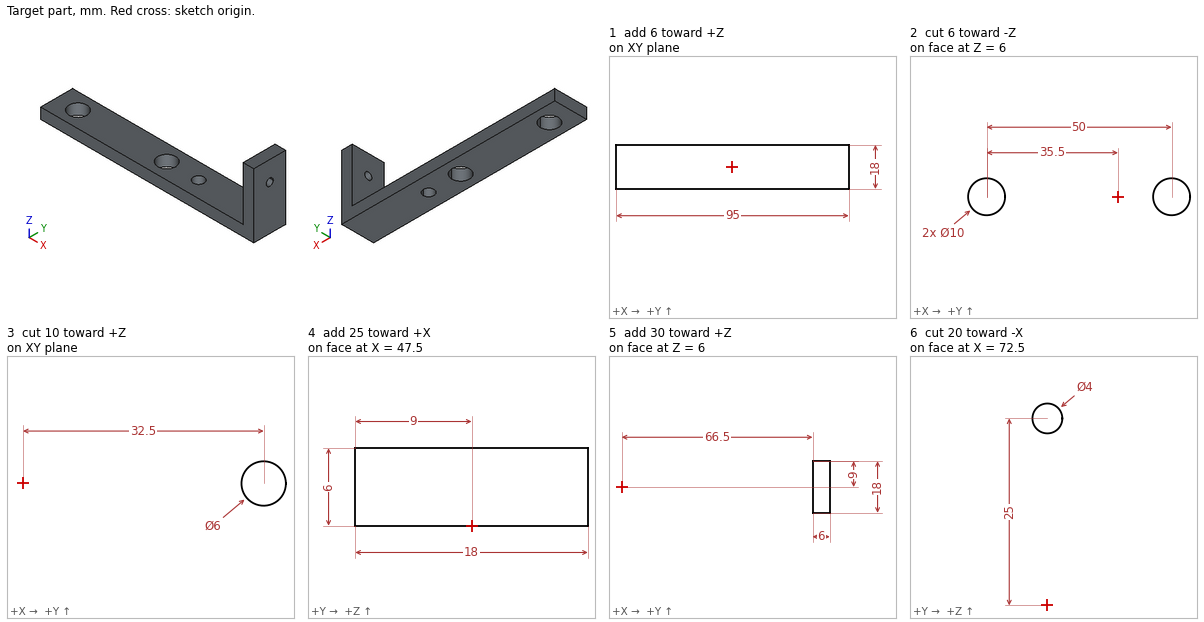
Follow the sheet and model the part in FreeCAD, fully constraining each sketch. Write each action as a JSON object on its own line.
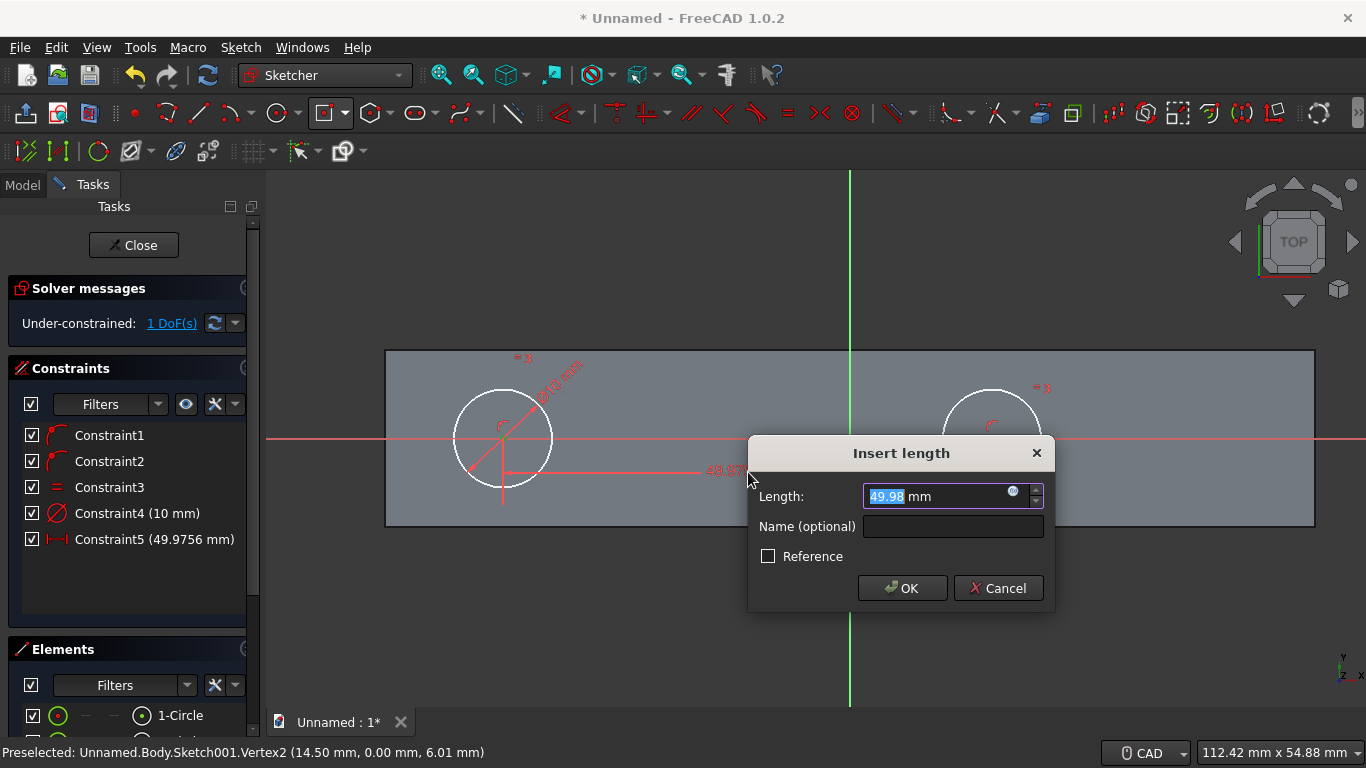
{"action": "type", "text": "50"}
{"action": "key", "text": "Return"}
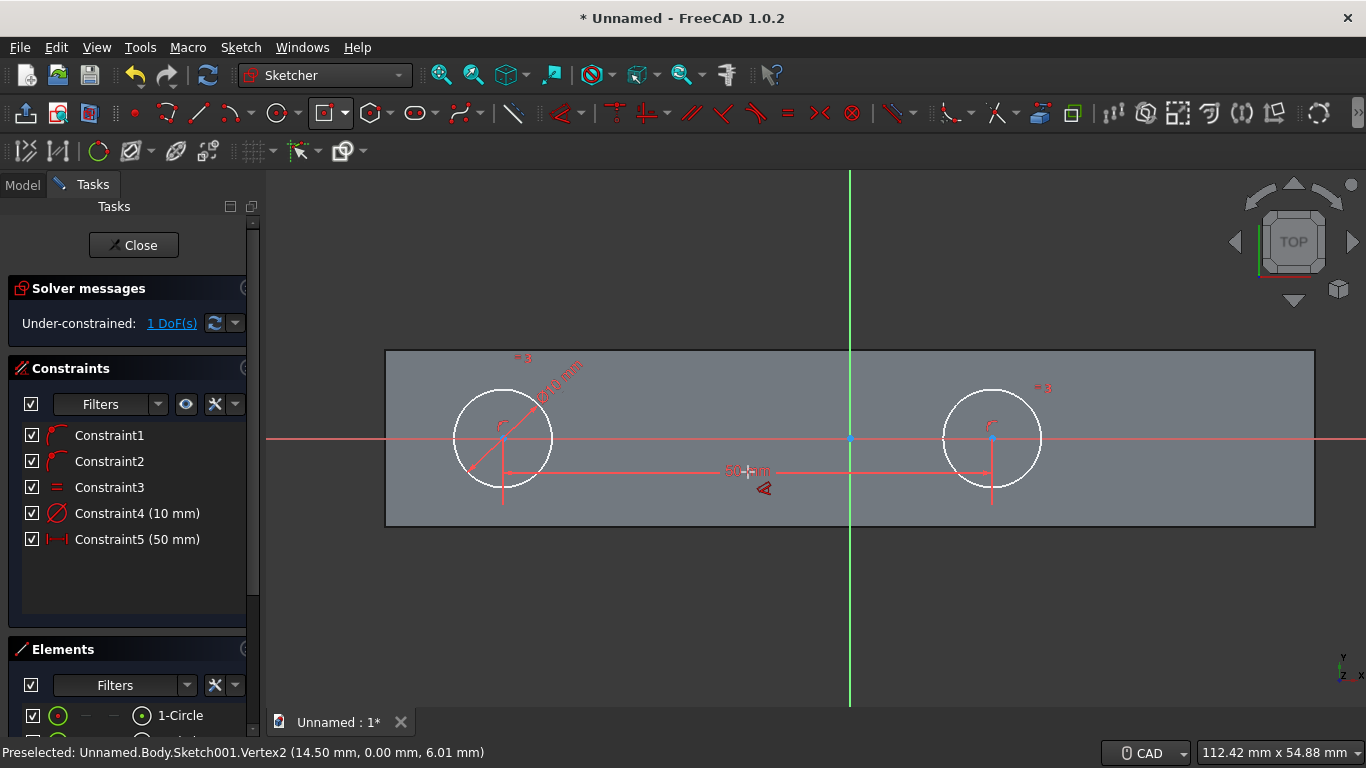
{"action": "left_click", "coordinate": [503, 438]}
{"action": "left_click", "coordinate": [677, 472]}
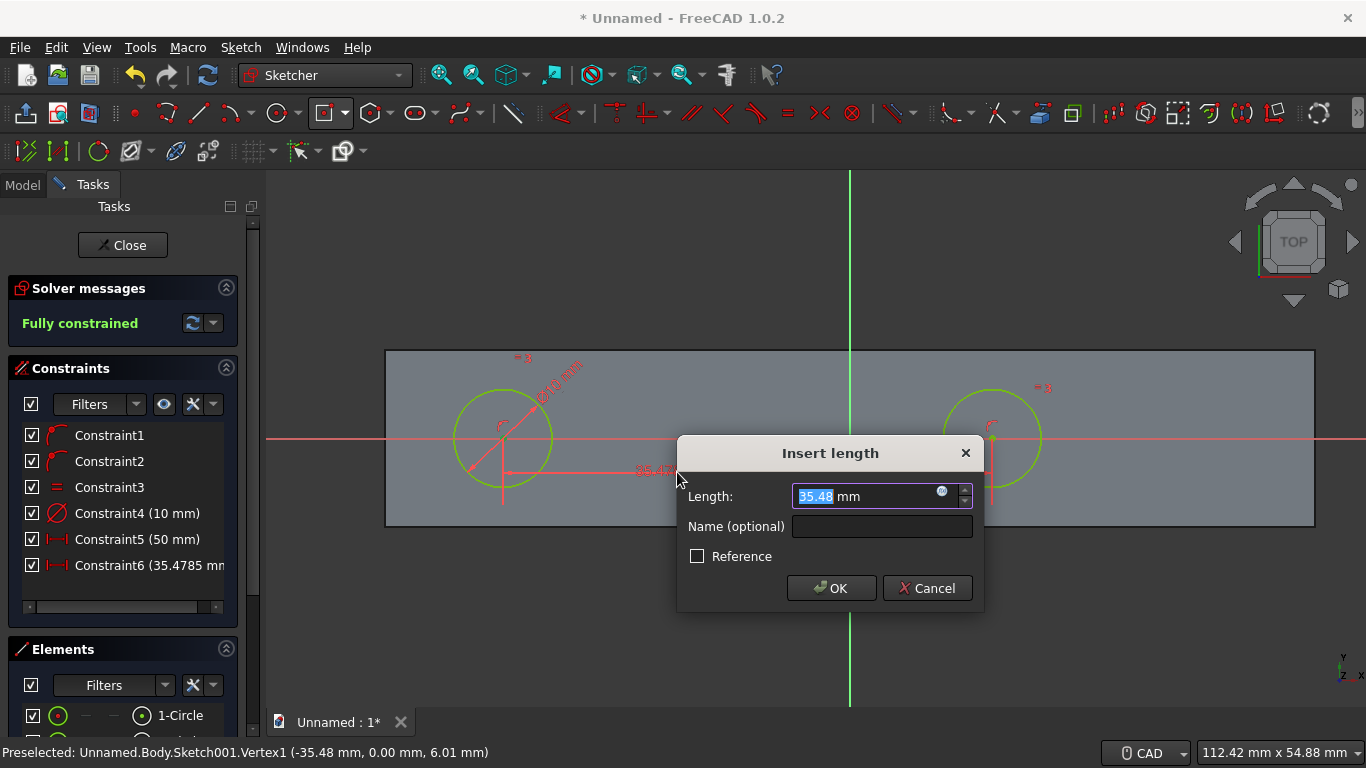
{"action": "type", "text": "35.5"}
{"action": "key", "text": "Return"}
{"action": "key", "text": "Escape"}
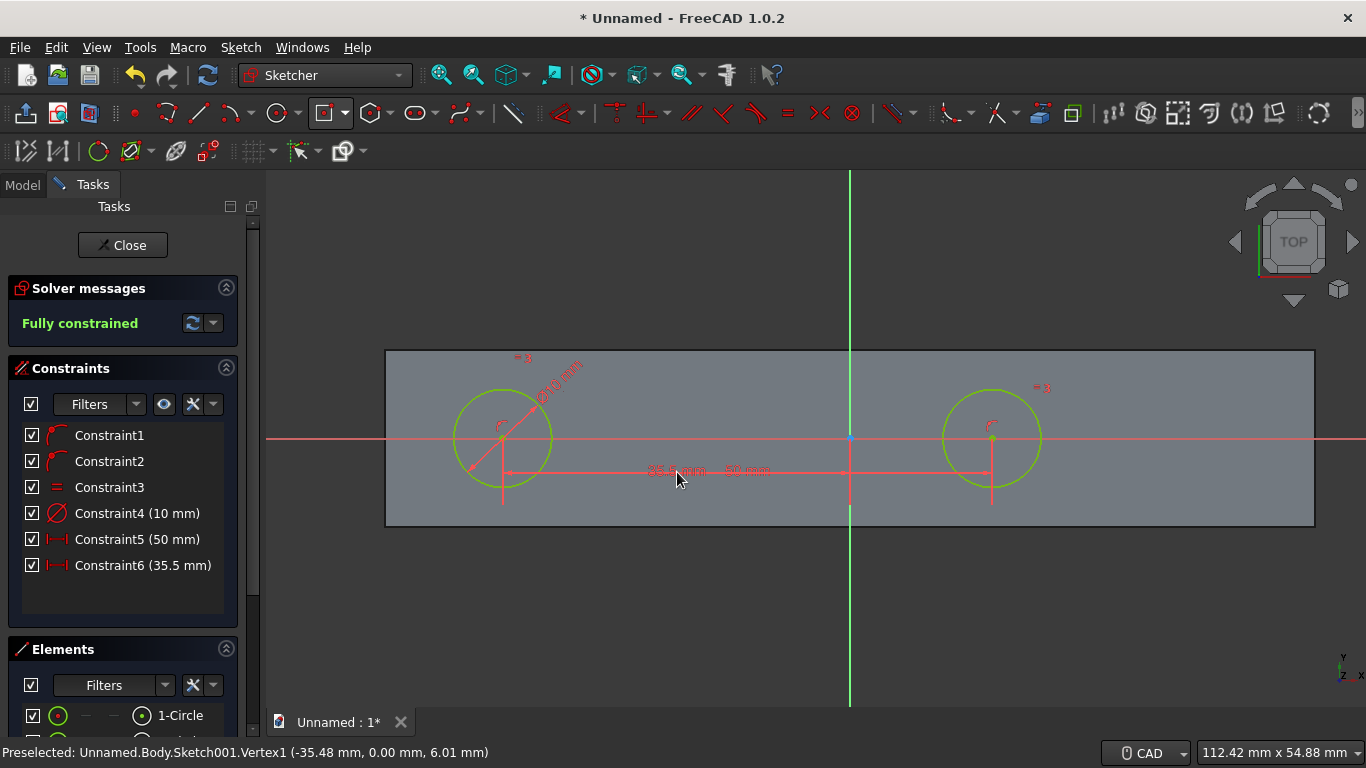
{"action": "left_click", "coordinate": [123, 245]}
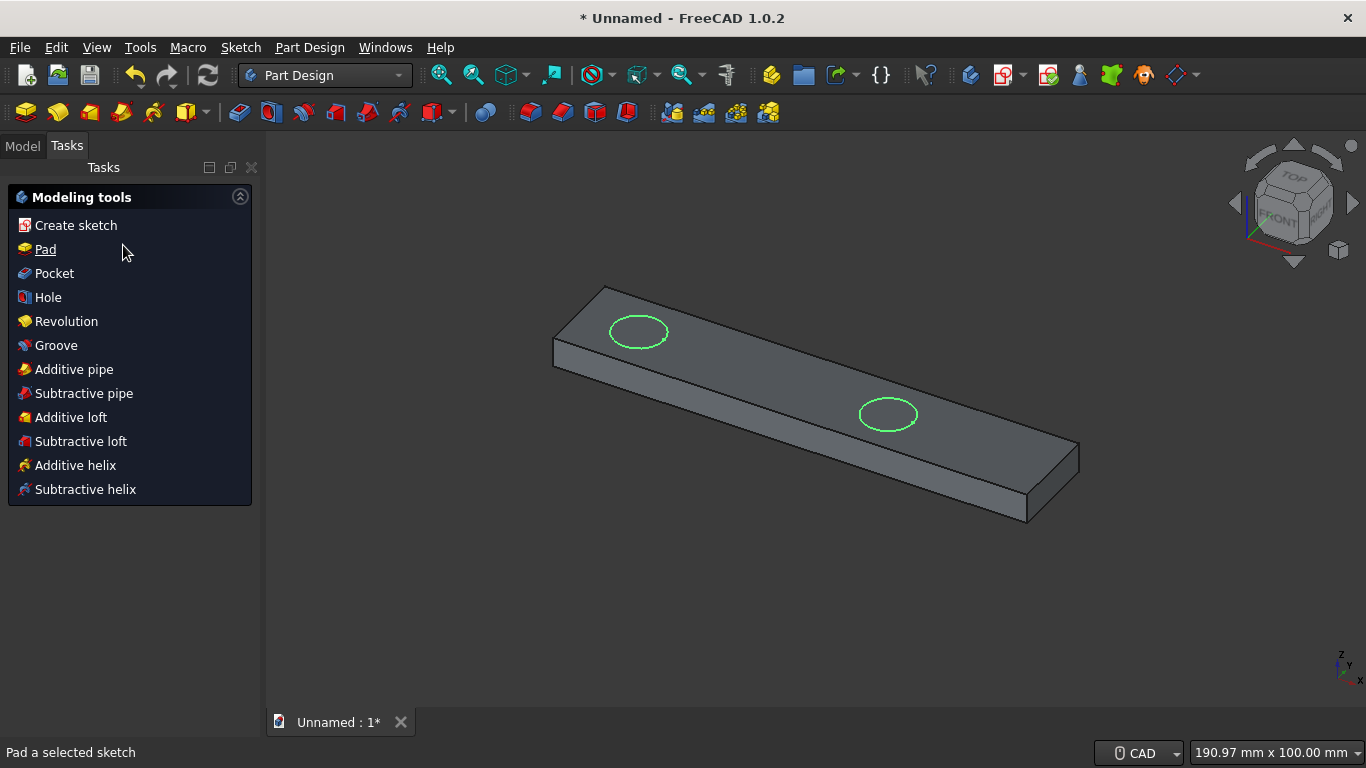
{"action": "left_click", "coordinate": [240, 112]}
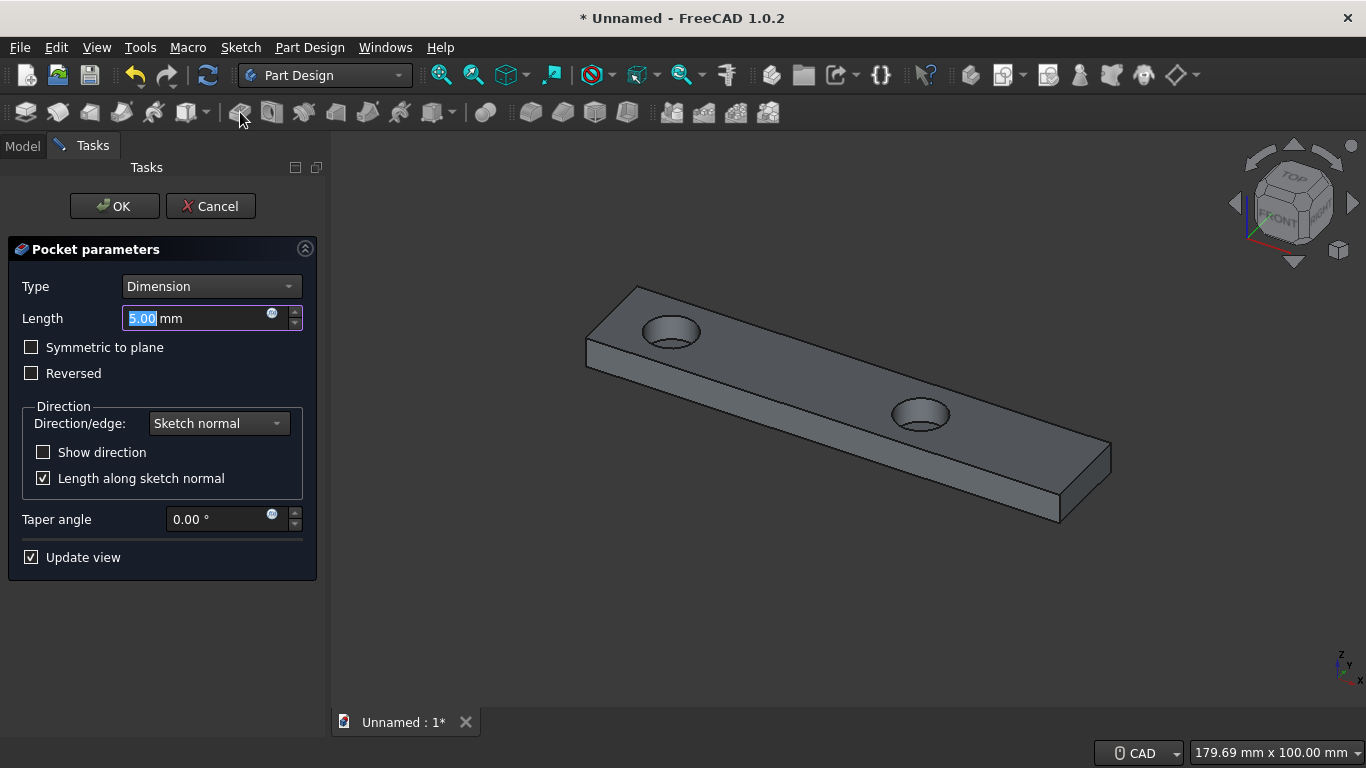
{"action": "type", "text": "6"}
{"action": "key", "text": "Tab"}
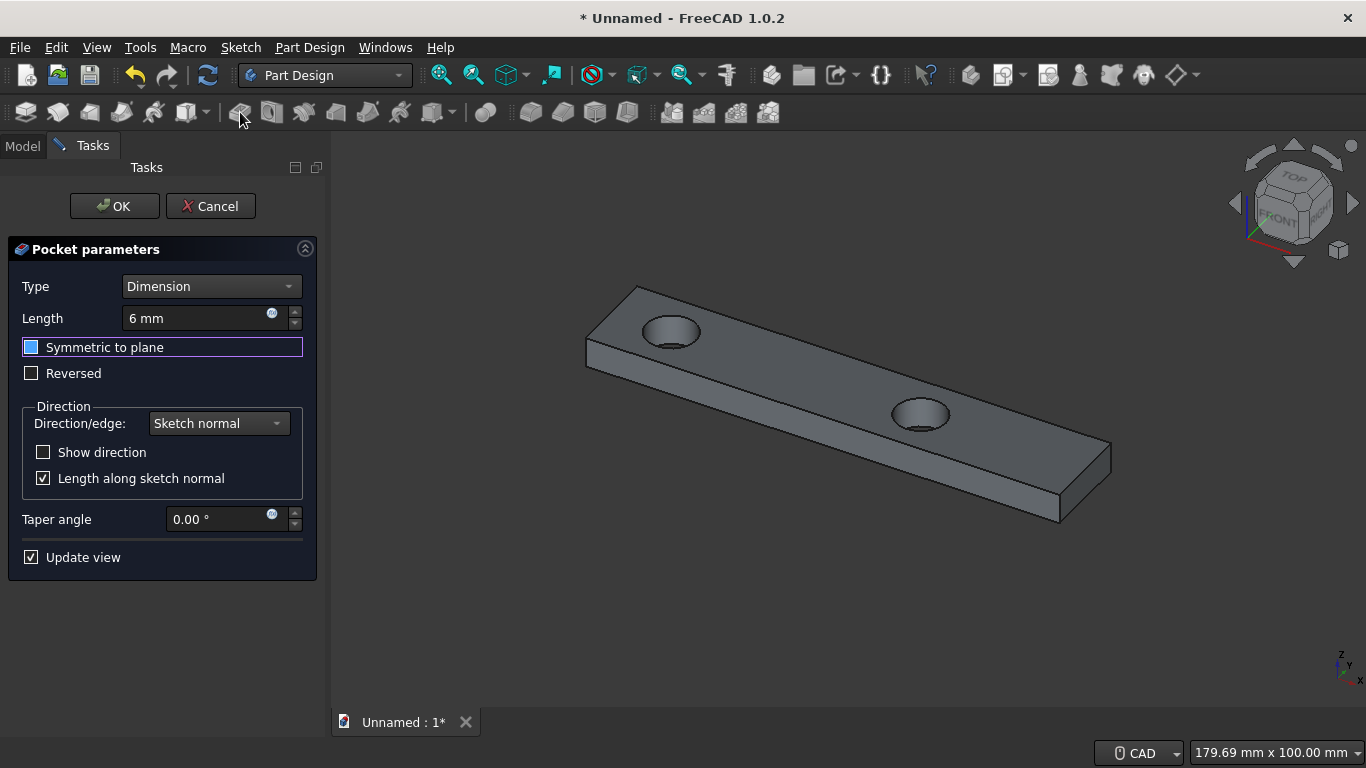
{"action": "left_click", "coordinate": [115, 206]}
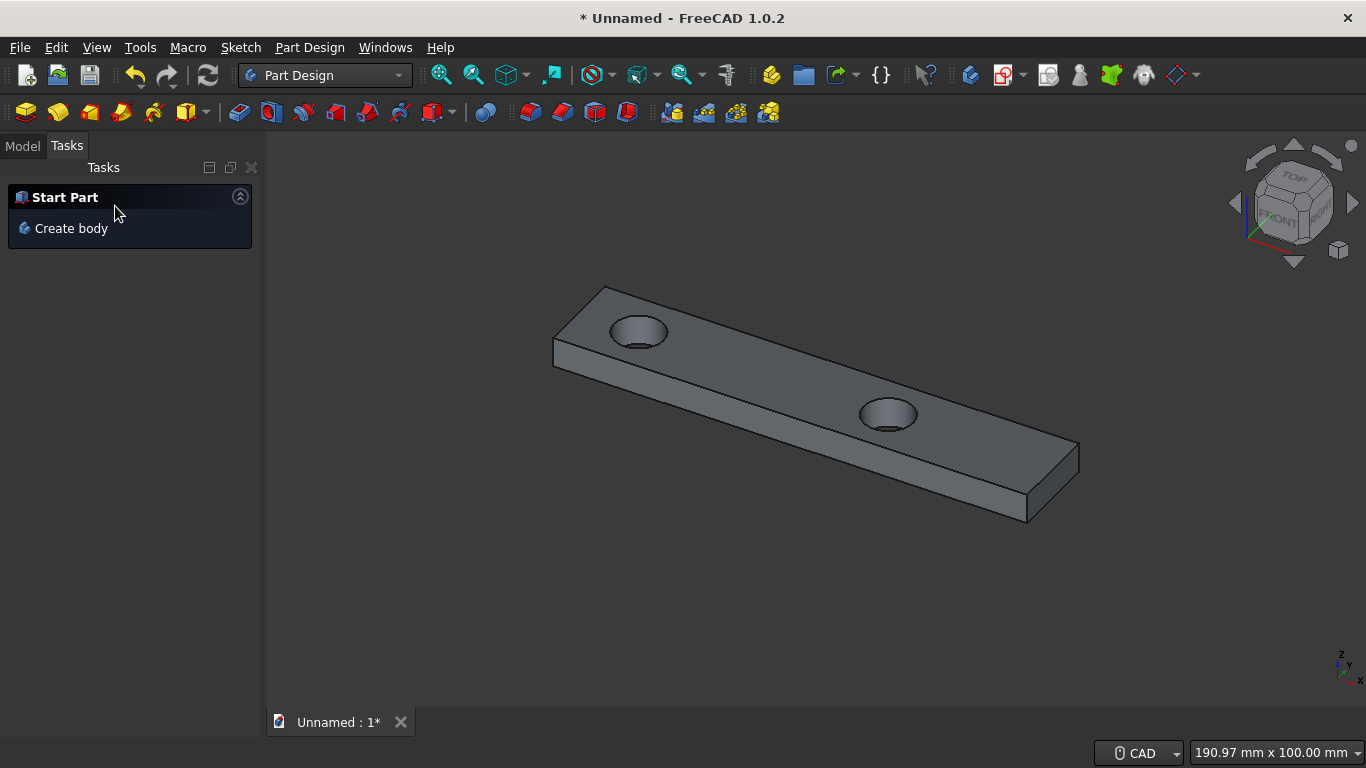
{"action": "left_click", "coordinate": [1004, 76]}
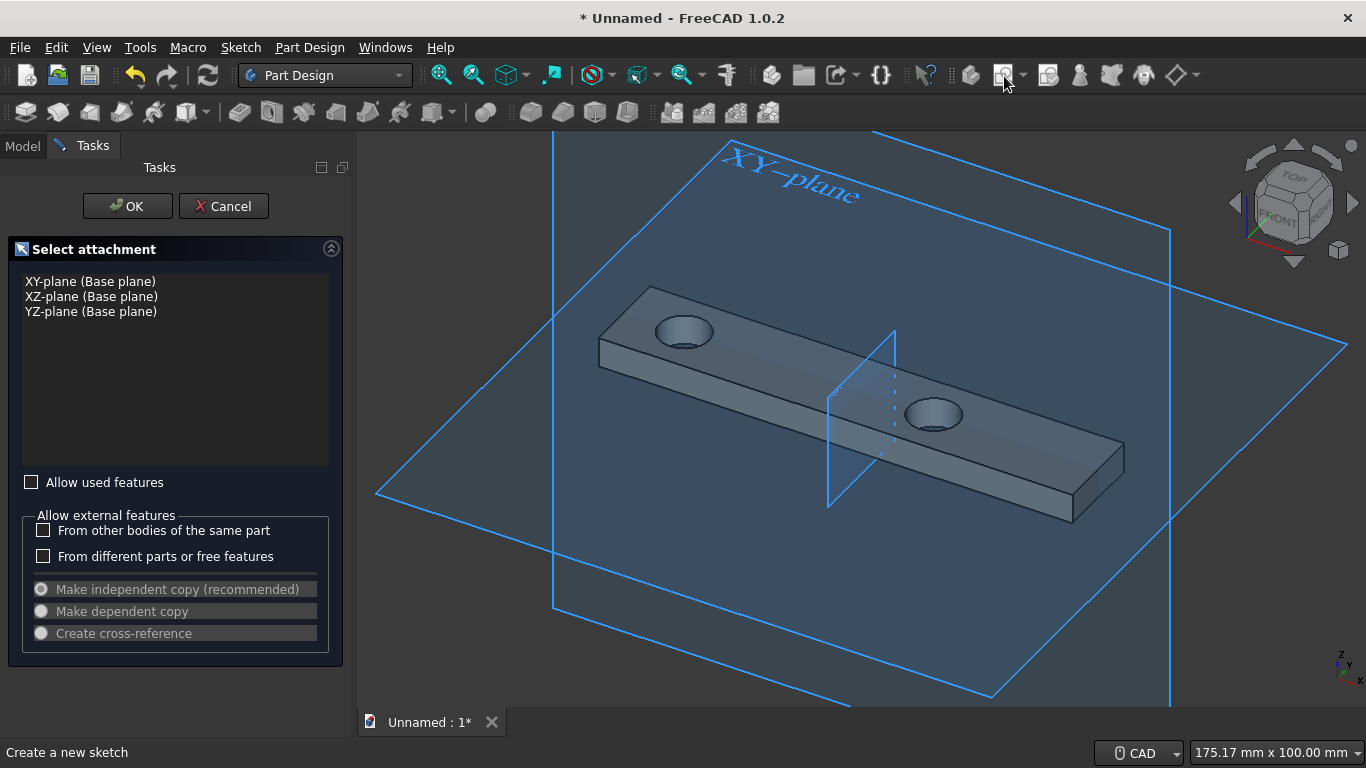
{"action": "left_click", "coordinate": [82, 282]}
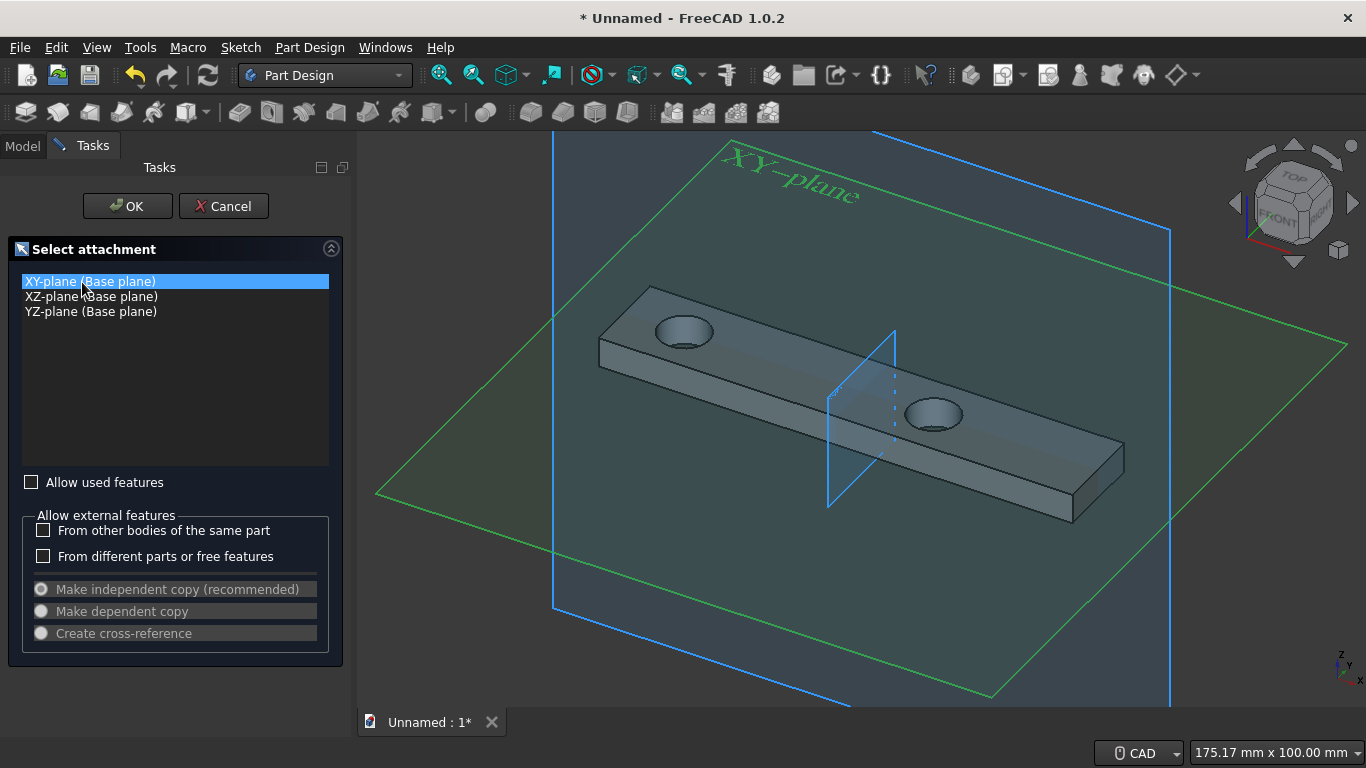
{"action": "left_click", "coordinate": [128, 206]}